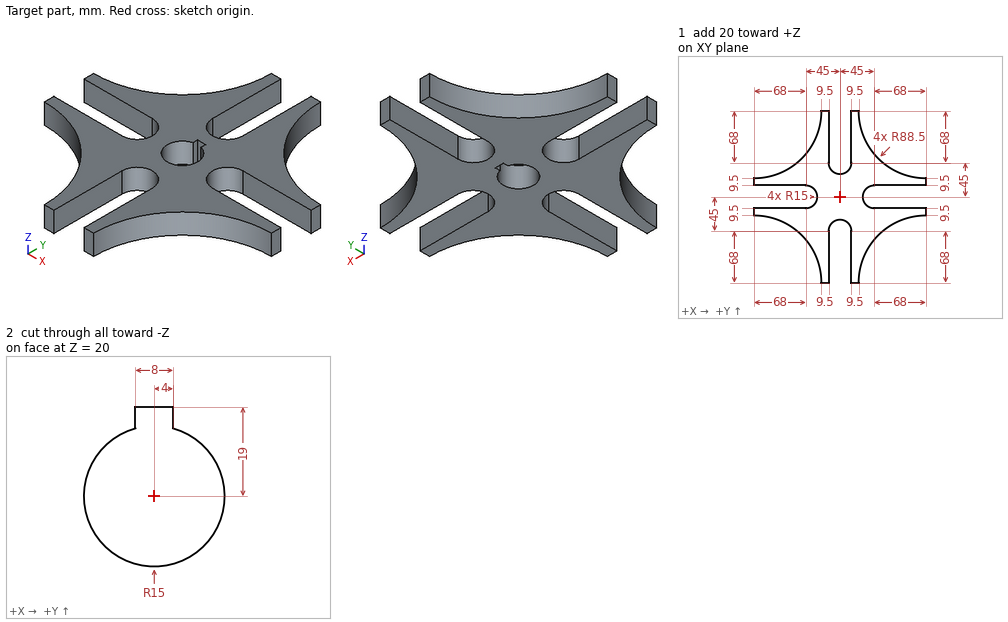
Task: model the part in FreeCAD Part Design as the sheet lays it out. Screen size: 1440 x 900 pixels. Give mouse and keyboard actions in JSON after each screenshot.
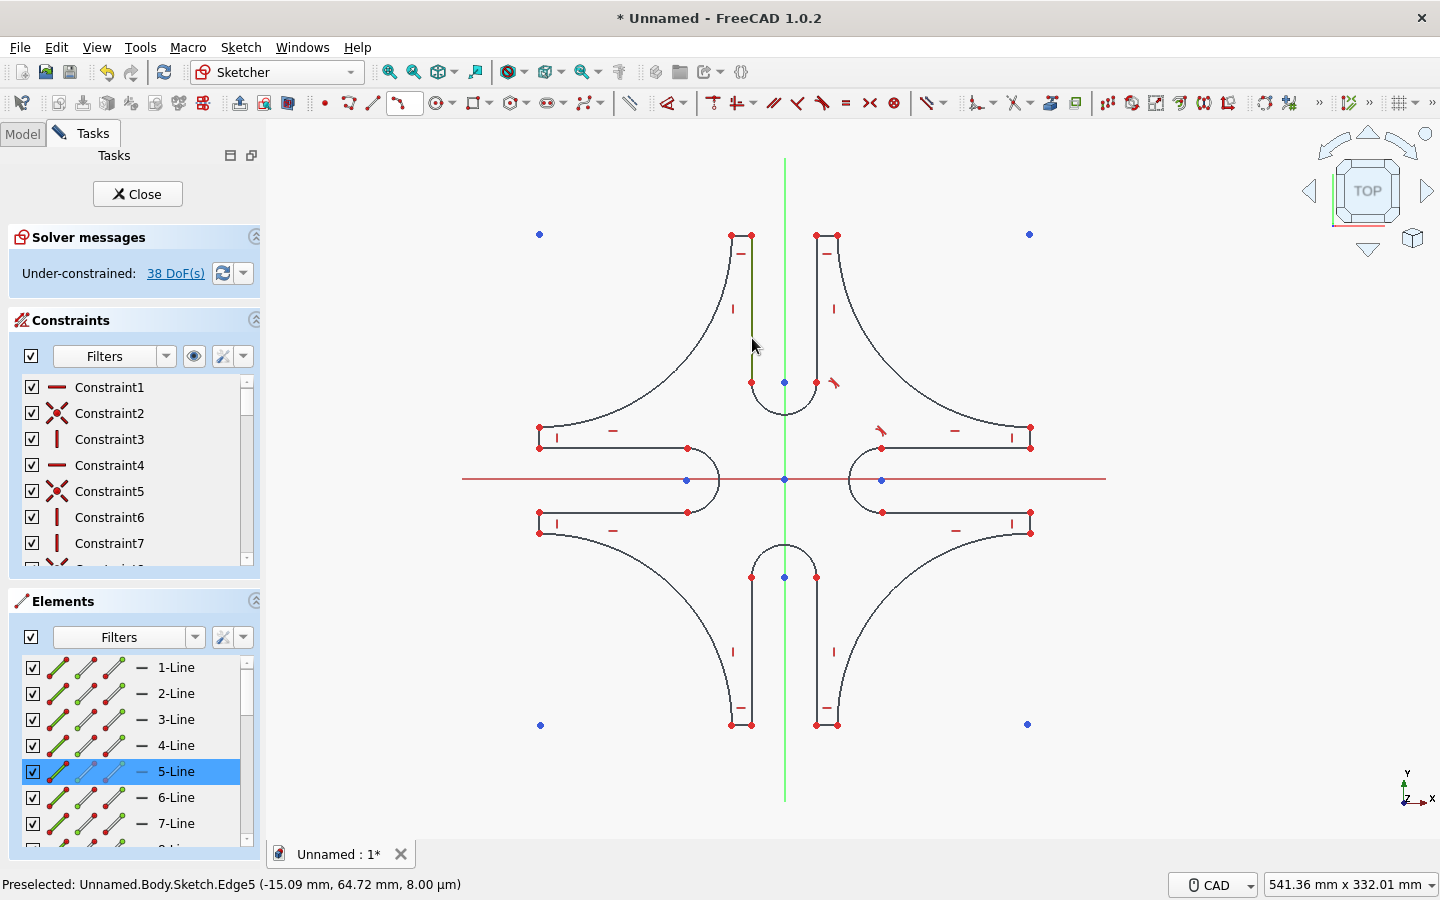
{"action": "left_click", "coordinate": [765, 408]}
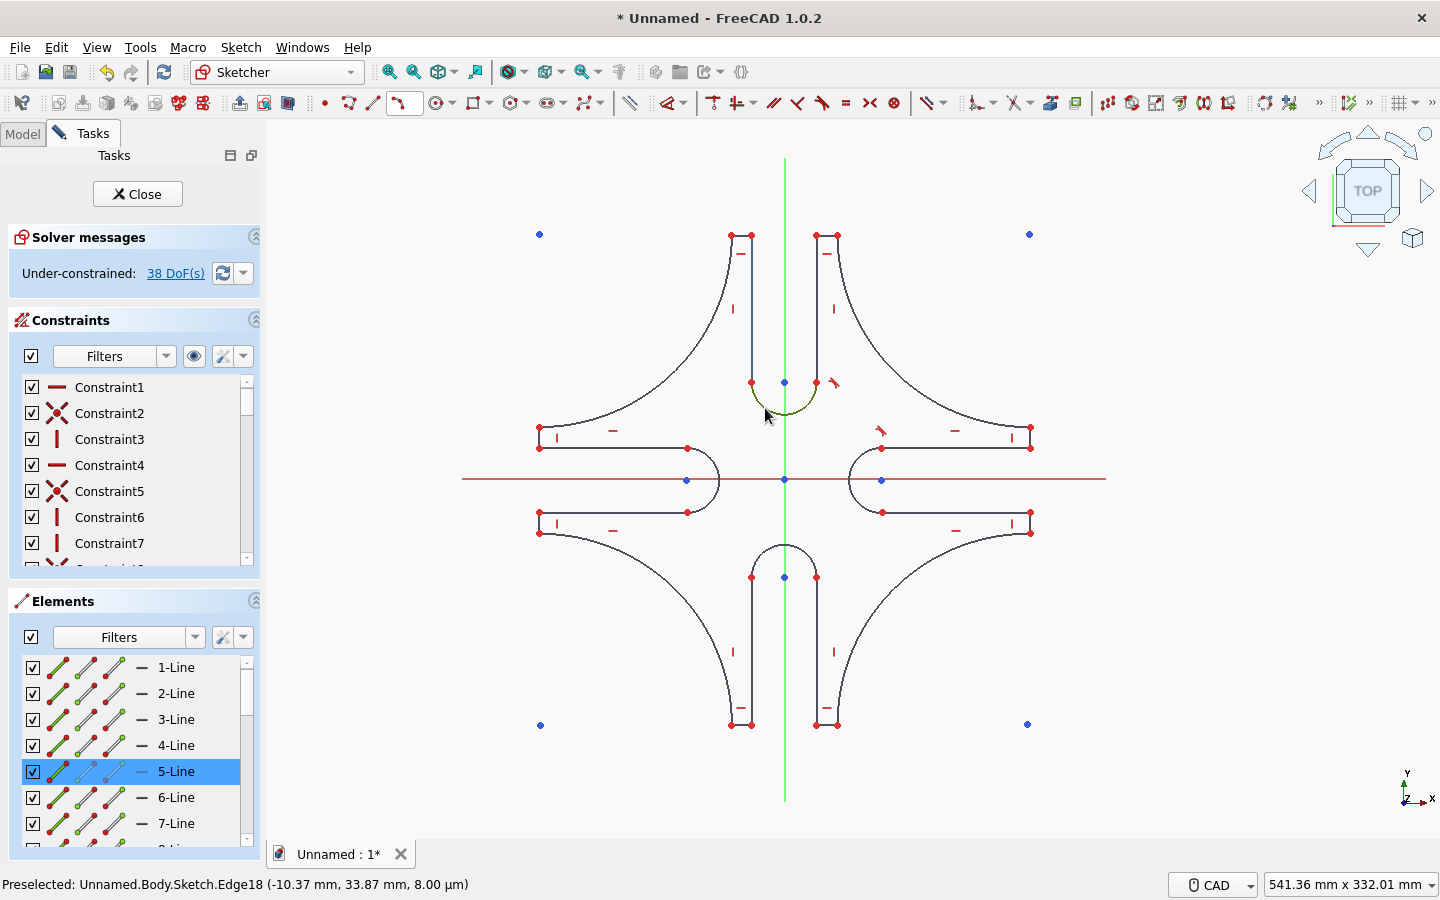
{"action": "left_click", "coordinate": [822, 104]}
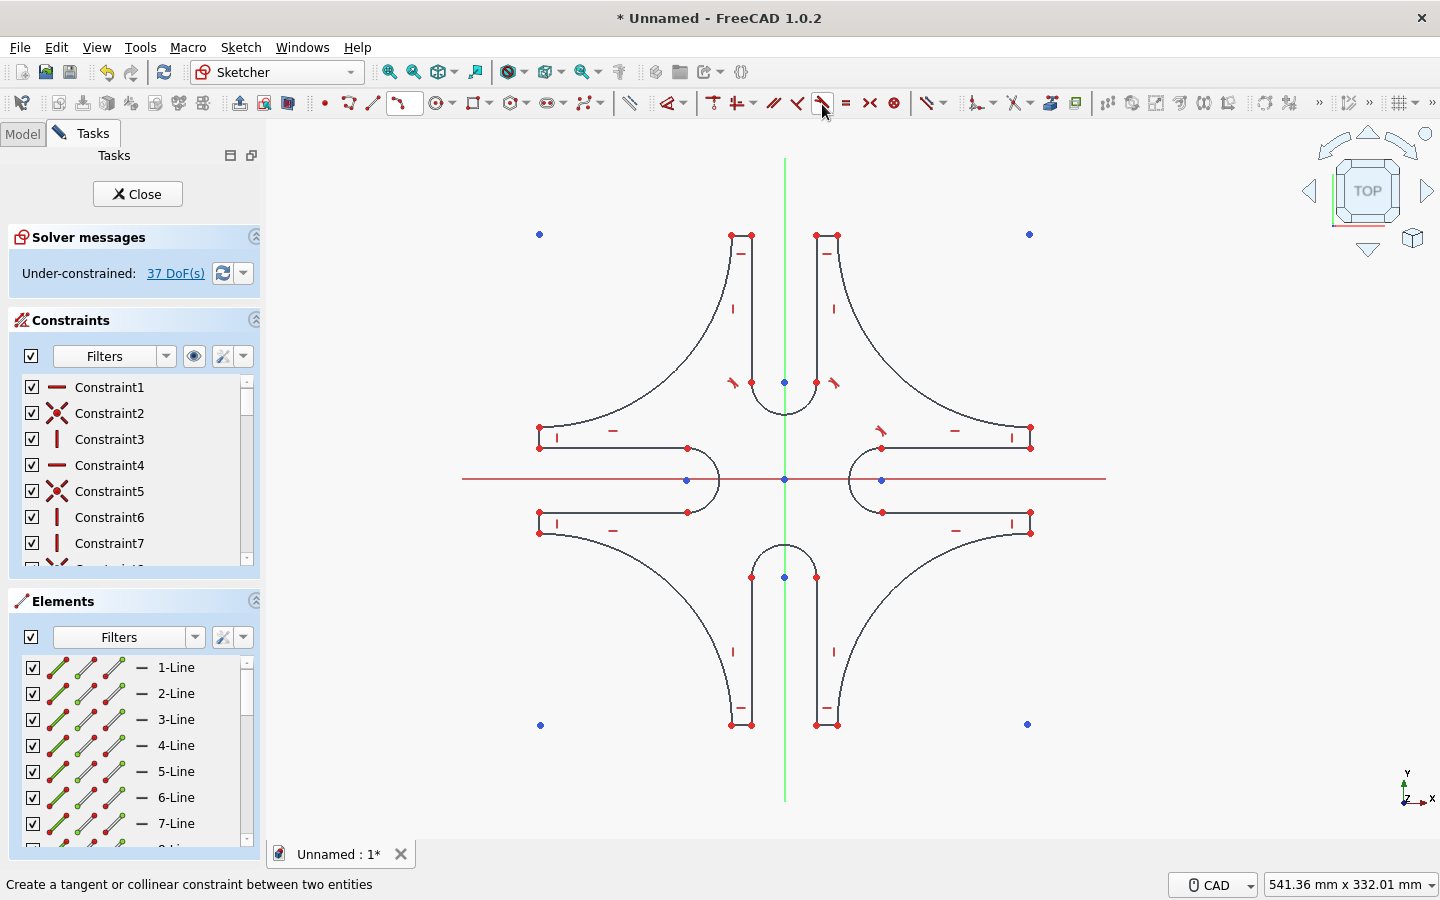
{"action": "left_click", "coordinate": [584, 448]}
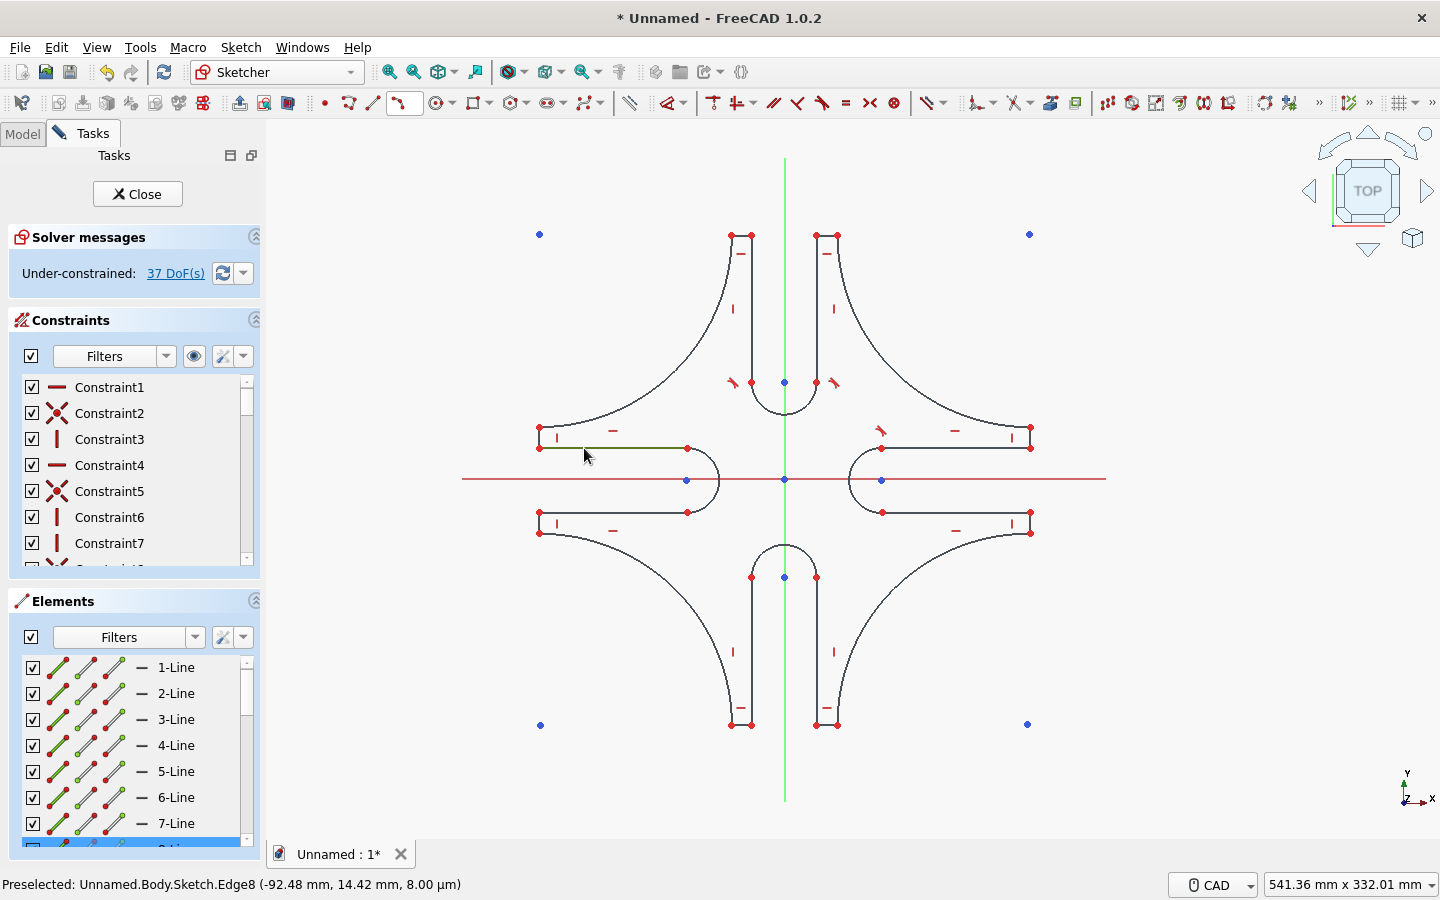
{"action": "left_click", "coordinate": [713, 499]}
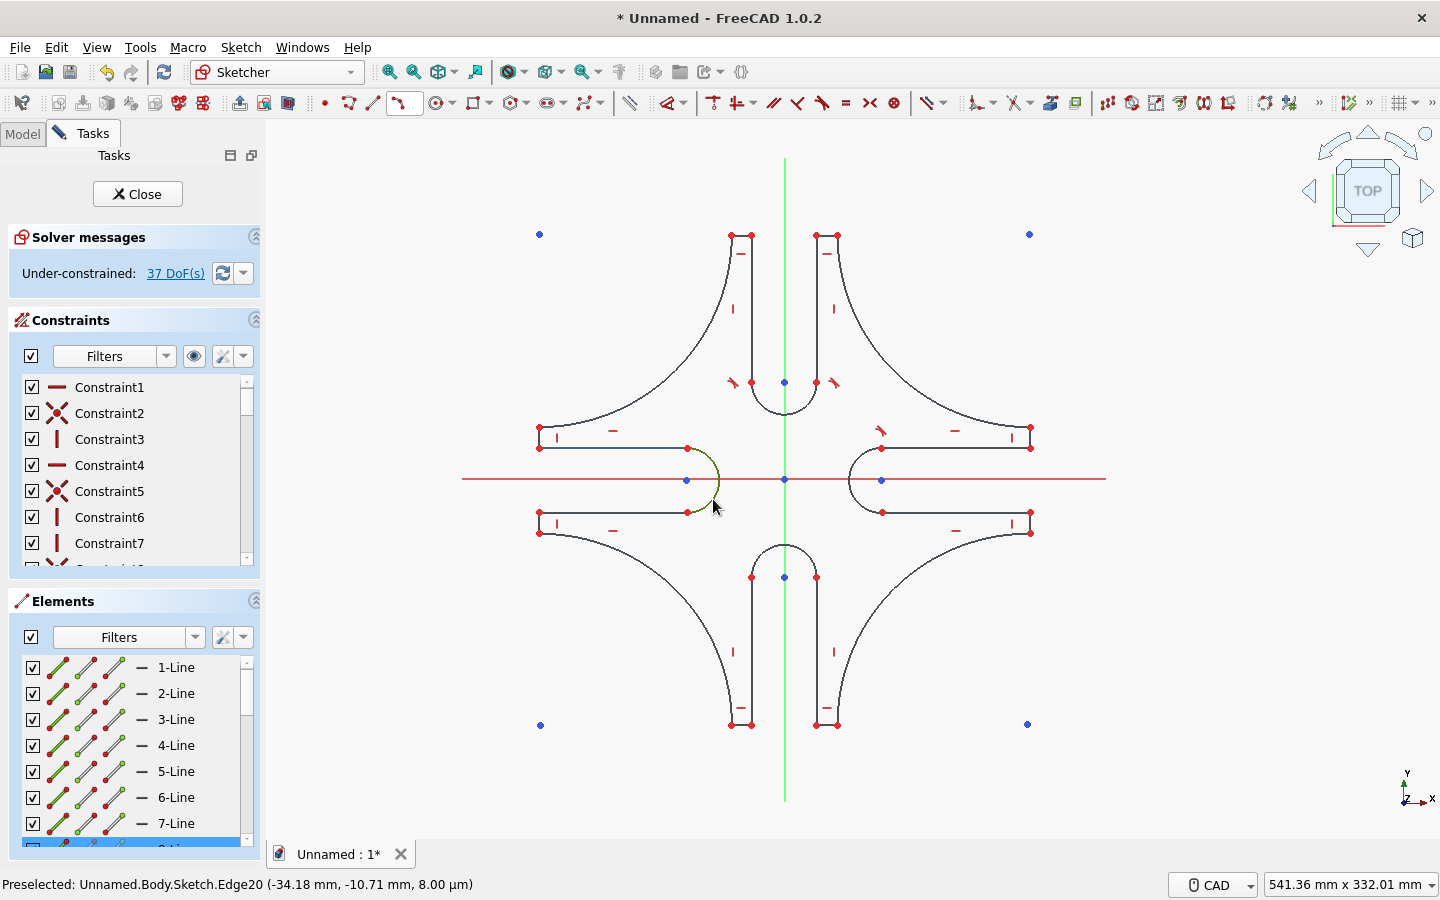
{"action": "left_click", "coordinate": [822, 104]}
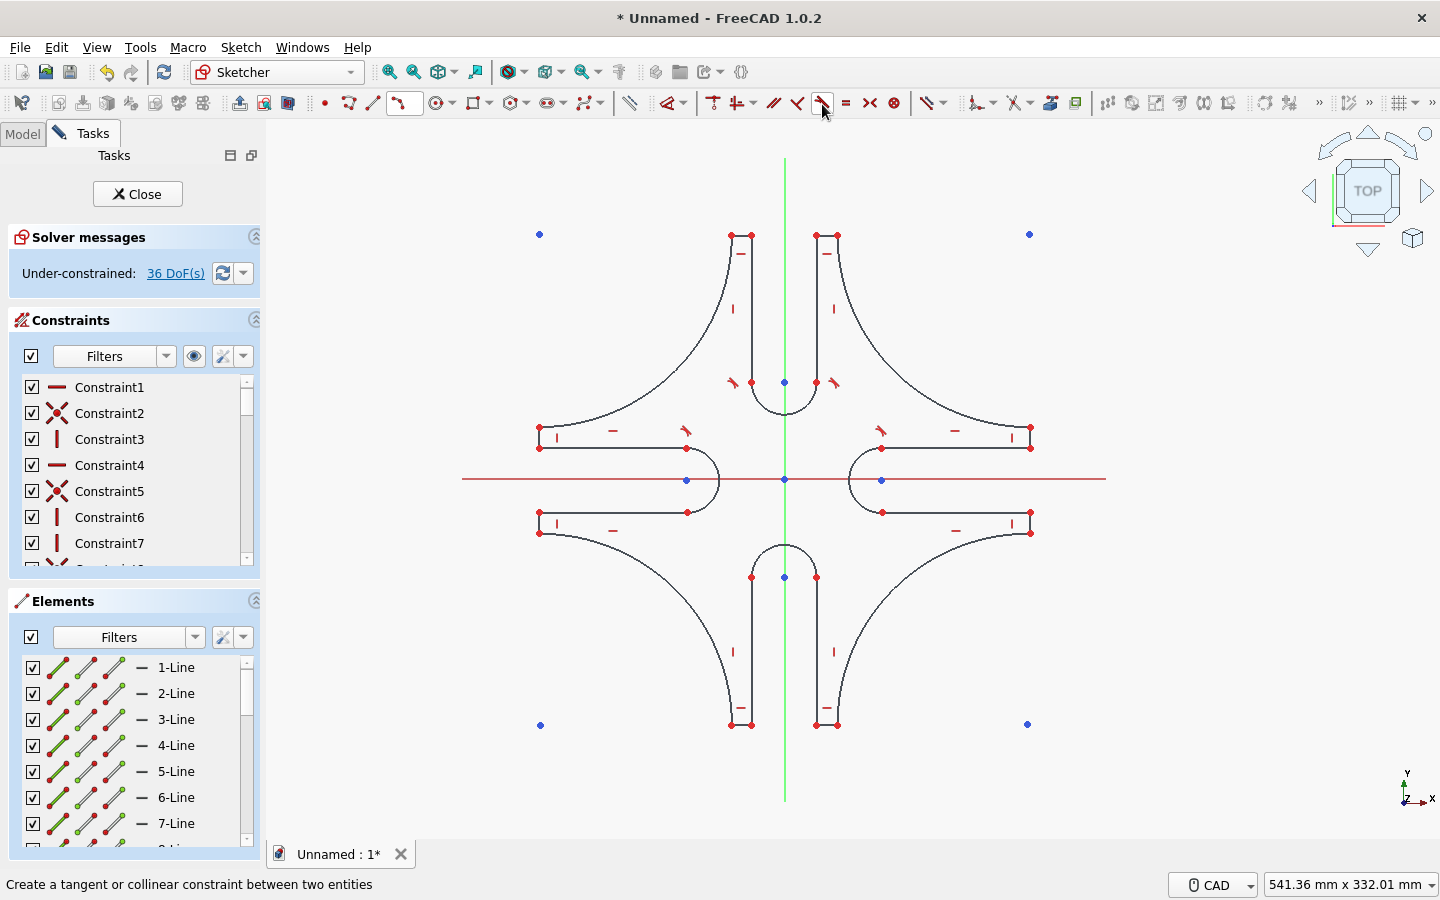
{"action": "left_click", "coordinate": [643, 513]}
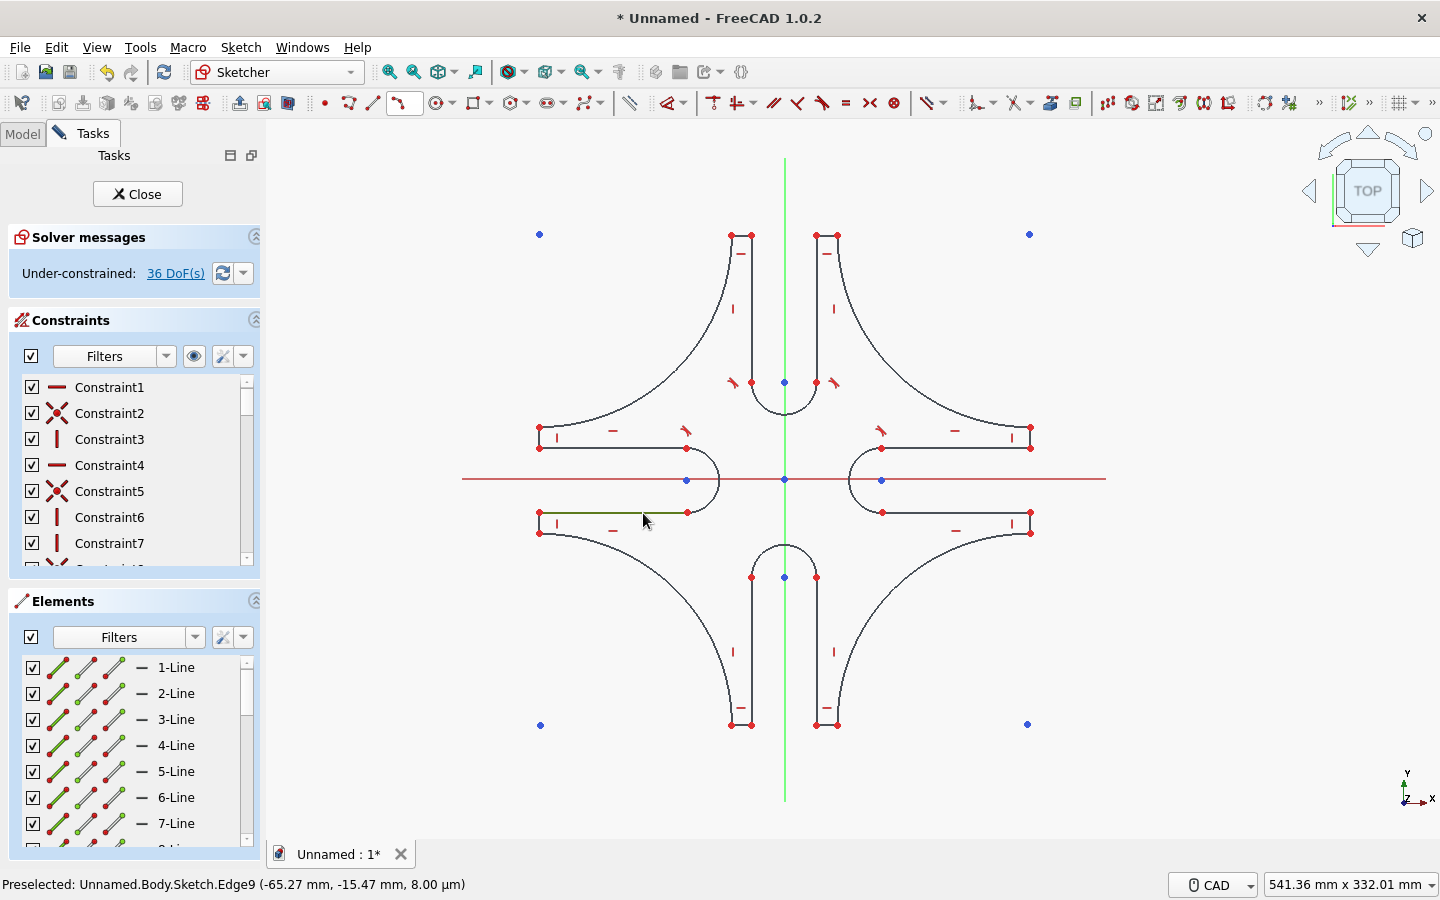
{"action": "left_click", "coordinate": [713, 499]}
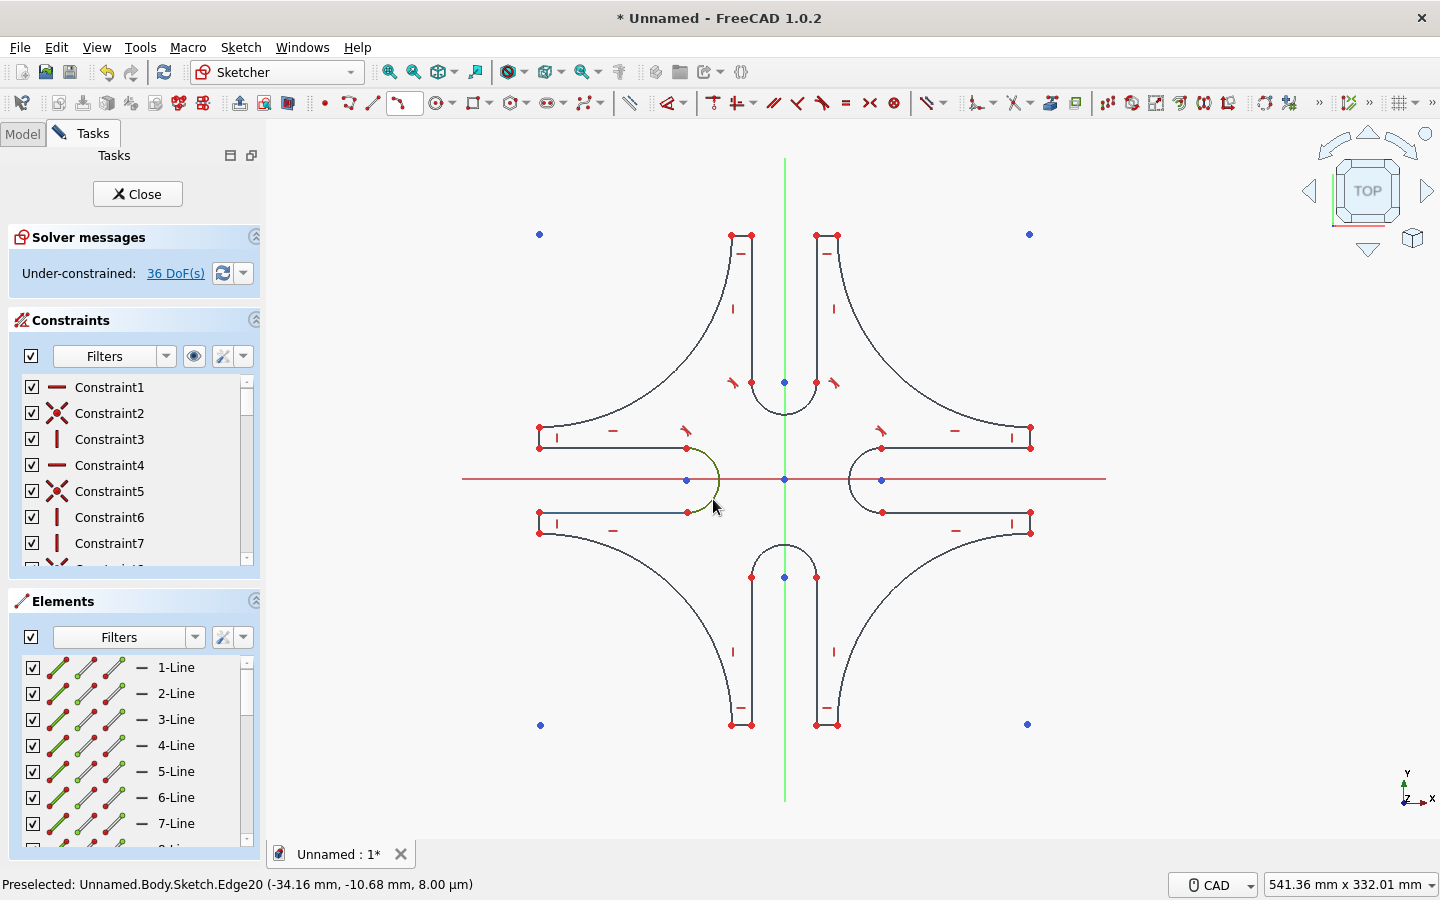
{"action": "left_click", "coordinate": [822, 104]}